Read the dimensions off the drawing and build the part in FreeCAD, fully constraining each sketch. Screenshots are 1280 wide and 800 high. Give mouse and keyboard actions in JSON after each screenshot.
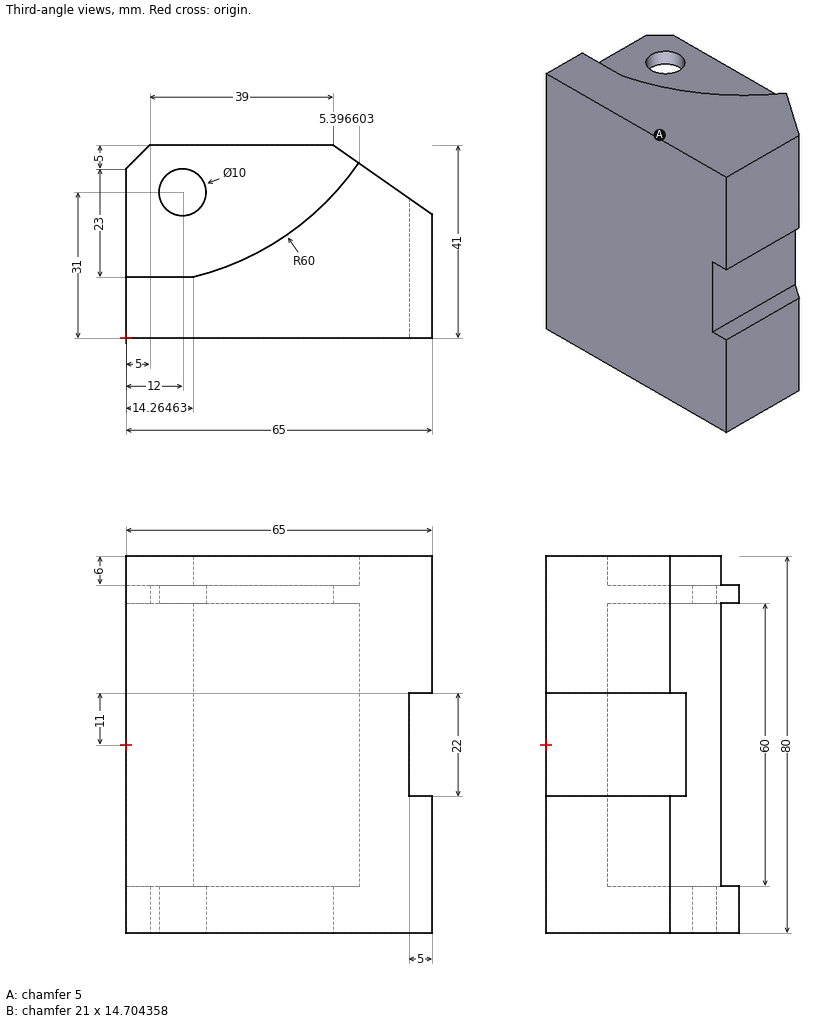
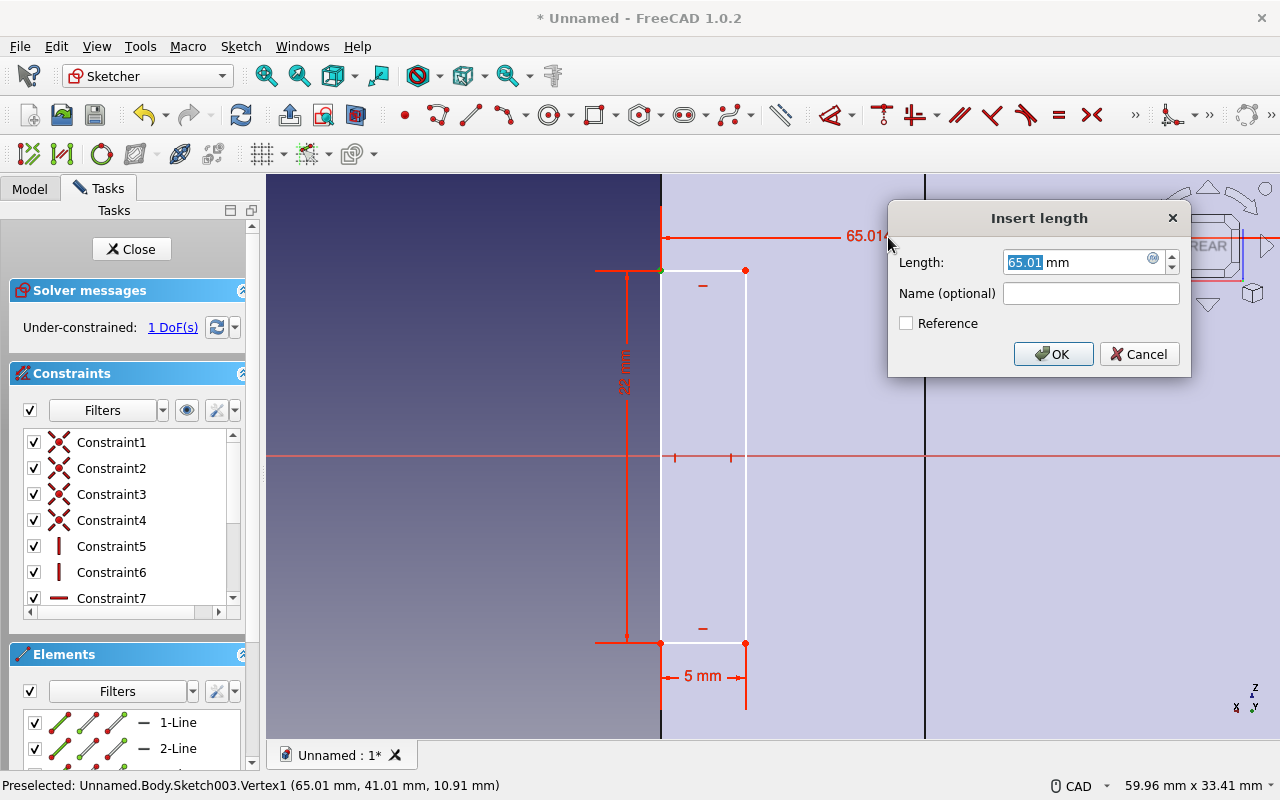
{"action": "type", "text": "65"}
{"action": "key", "text": "Return"}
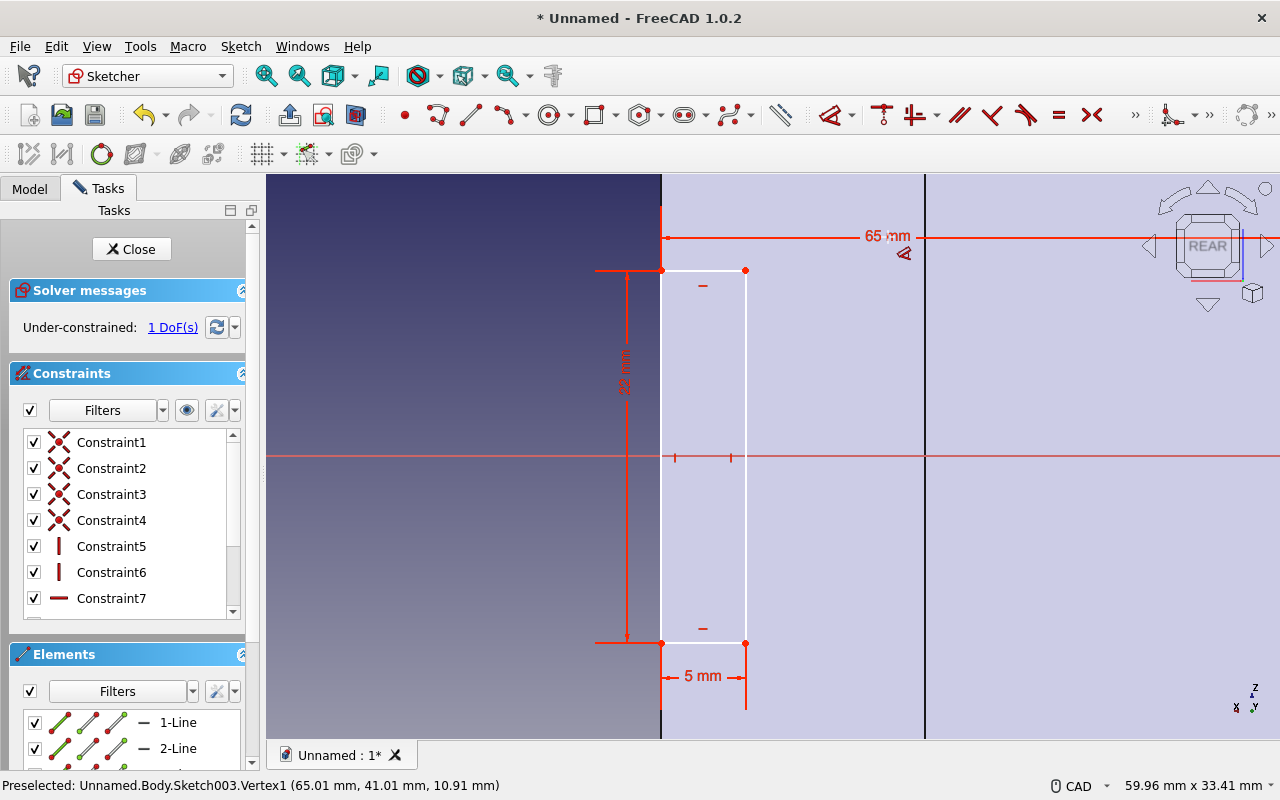
{"action": "left_click", "coordinate": [661, 271]}
{"action": "left_click", "coordinate": [627, 321]}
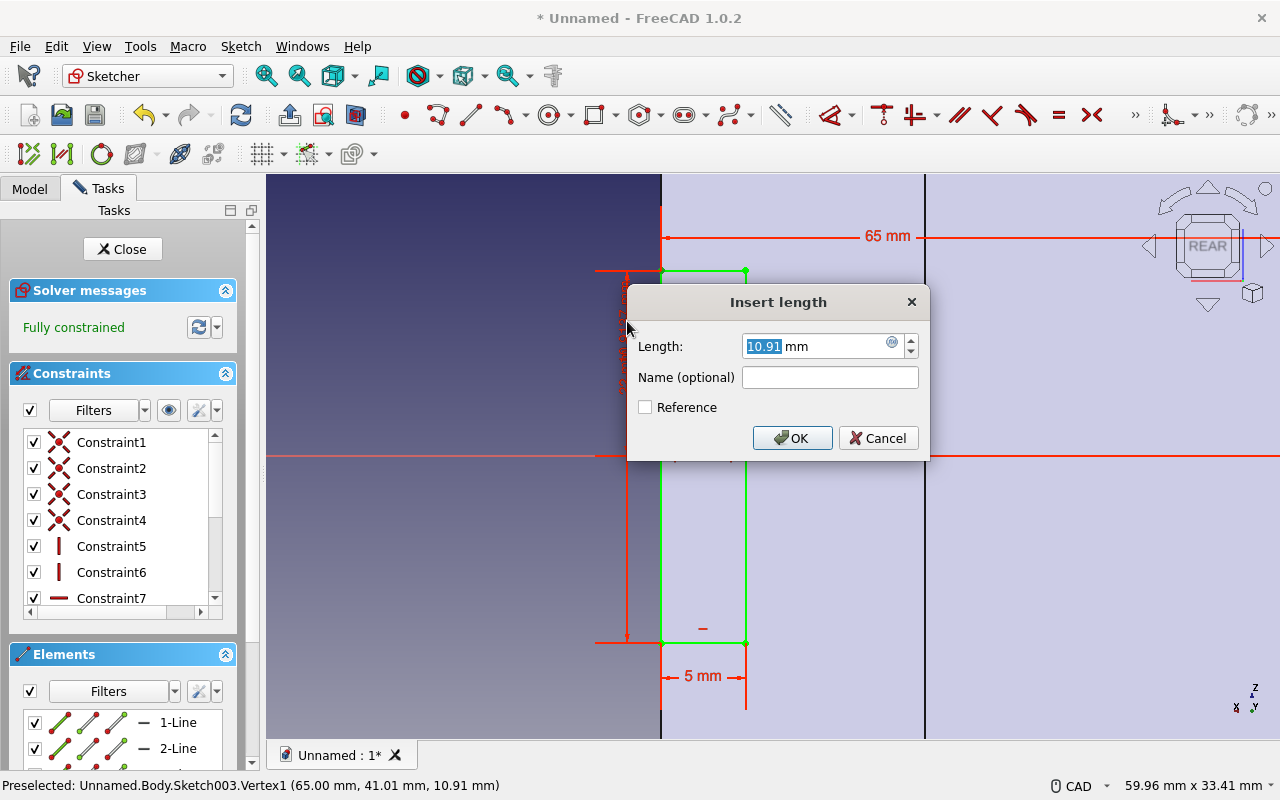
{"action": "type", "text": "11"}
{"action": "key", "text": "Return"}
{"action": "key", "text": "Escape"}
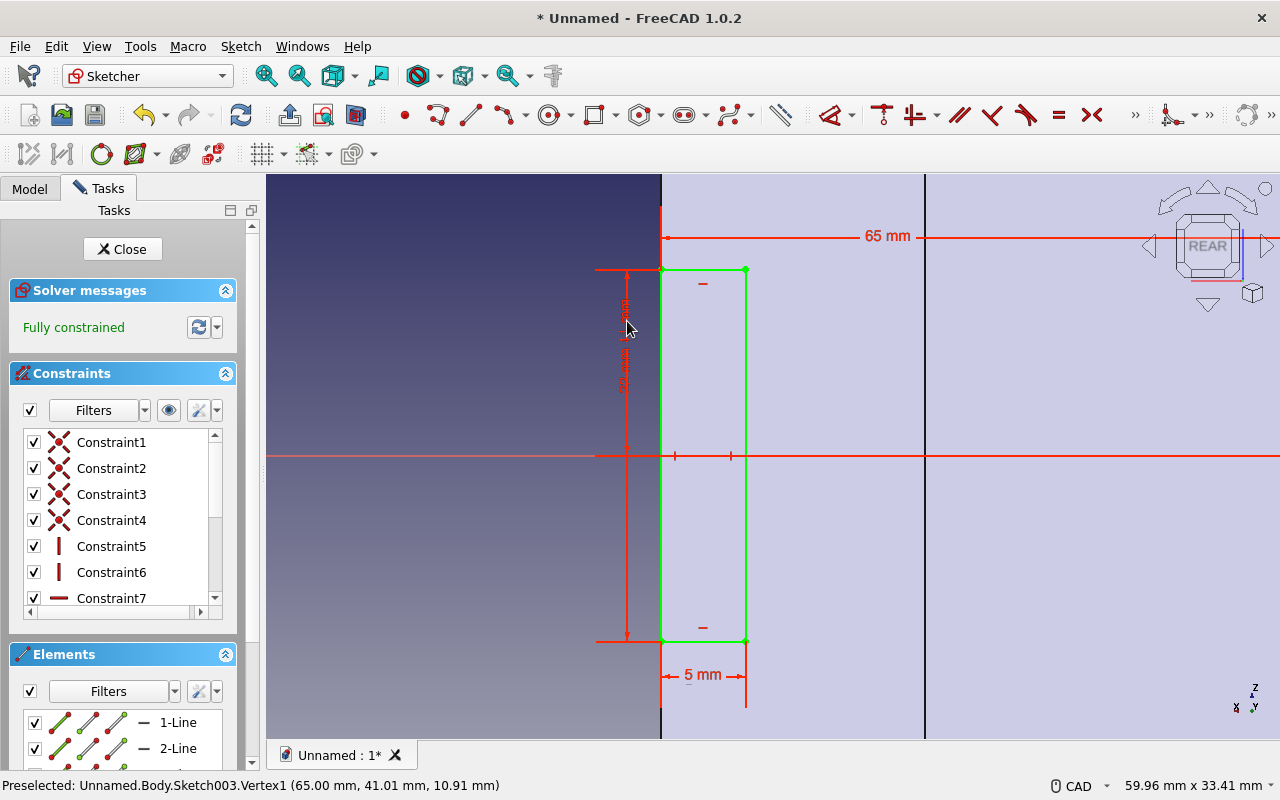
{"action": "left_click", "coordinate": [123, 249]}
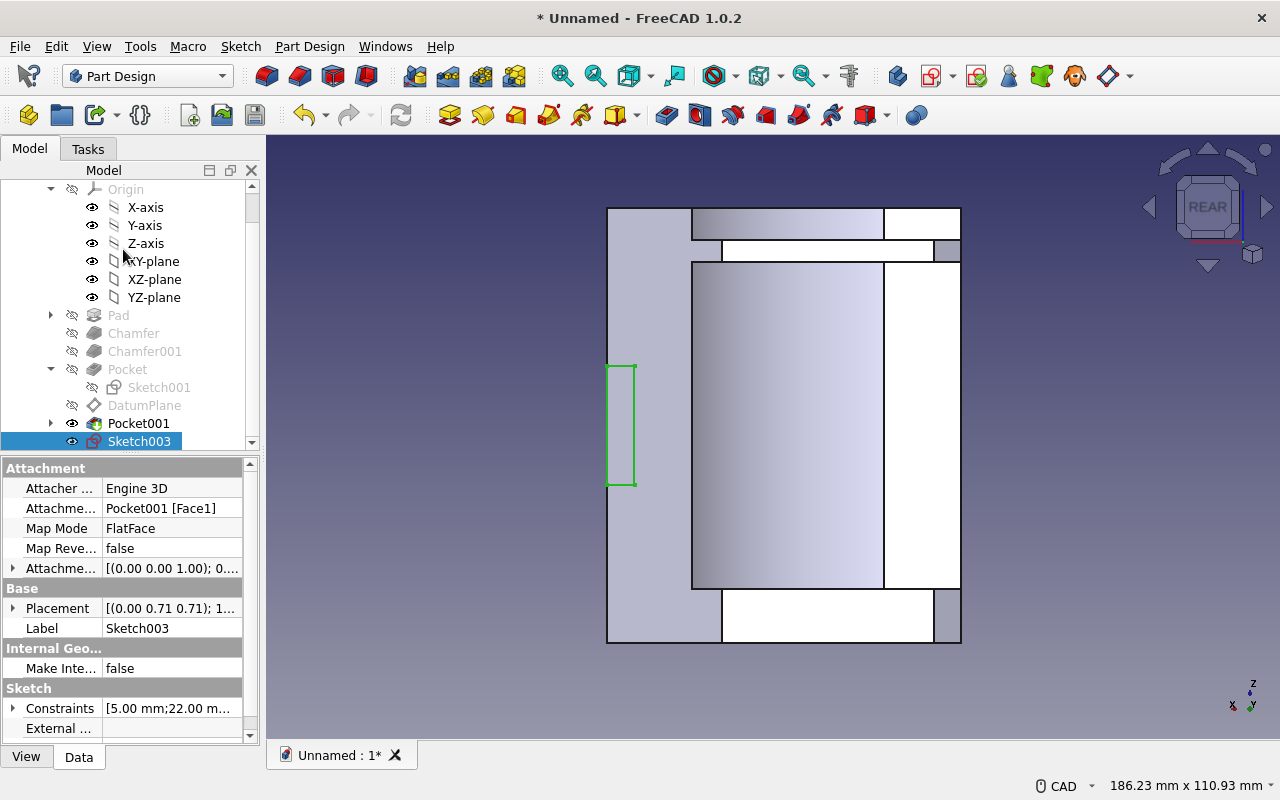
{"action": "left_click", "coordinate": [667, 116]}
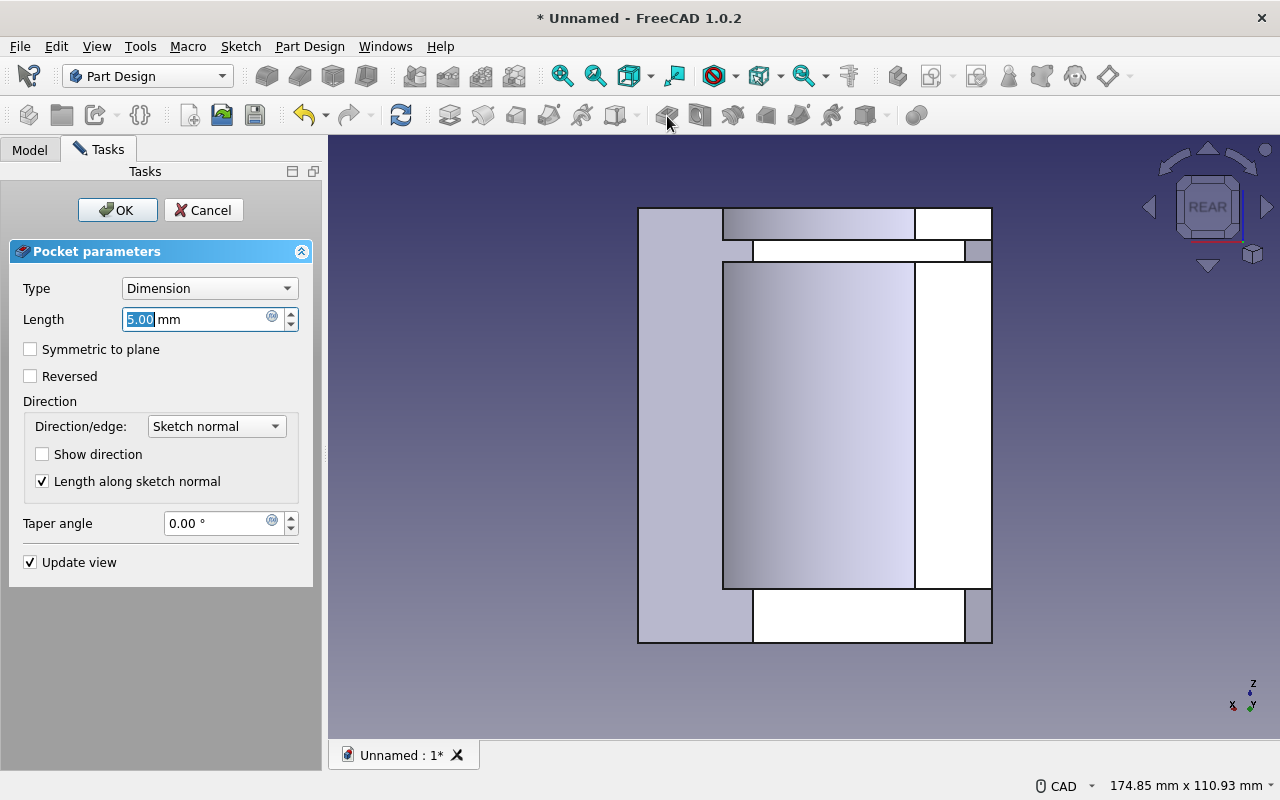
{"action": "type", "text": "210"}
{"action": "key", "text": "Tab"}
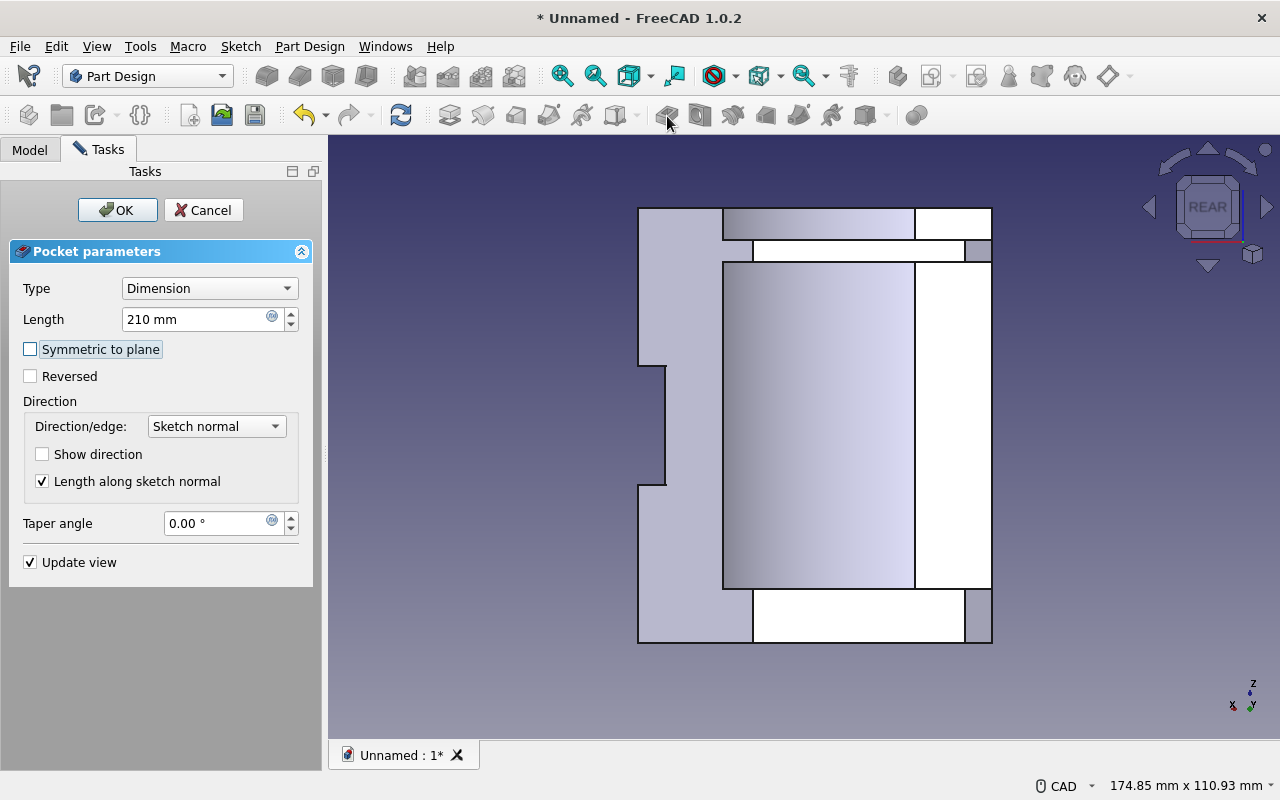
{"action": "left_click", "coordinate": [118, 210]}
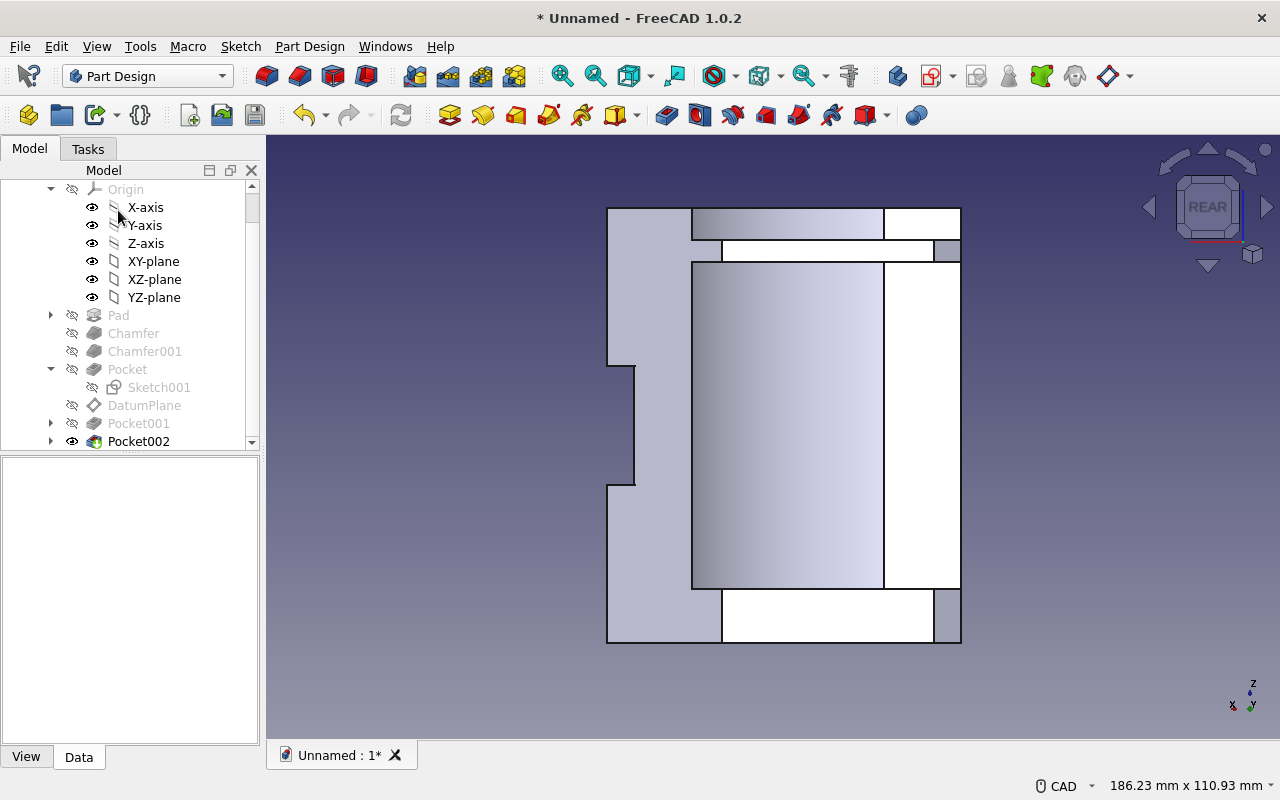
{"action": "key", "text": "0"}